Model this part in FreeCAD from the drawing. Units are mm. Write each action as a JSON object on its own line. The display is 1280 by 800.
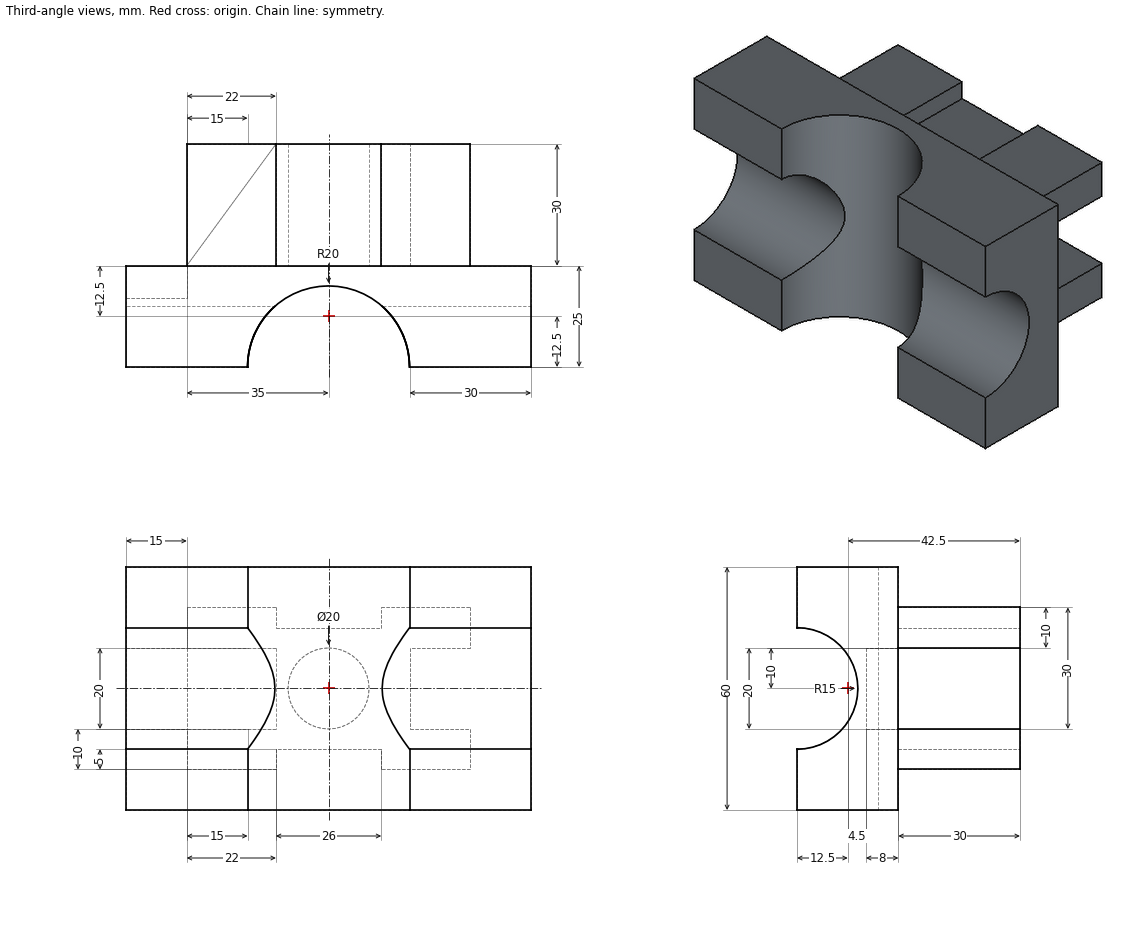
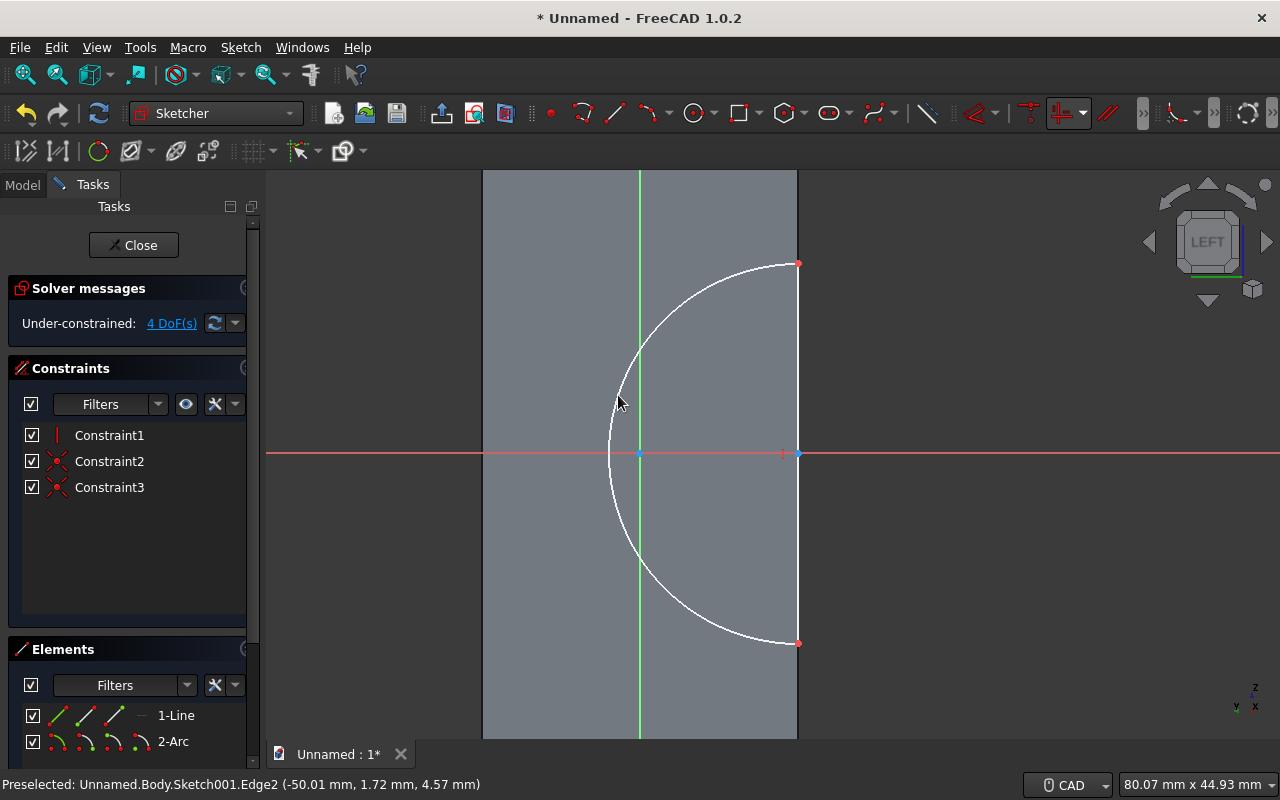
{"action": "left_click", "coordinate": [799, 454]}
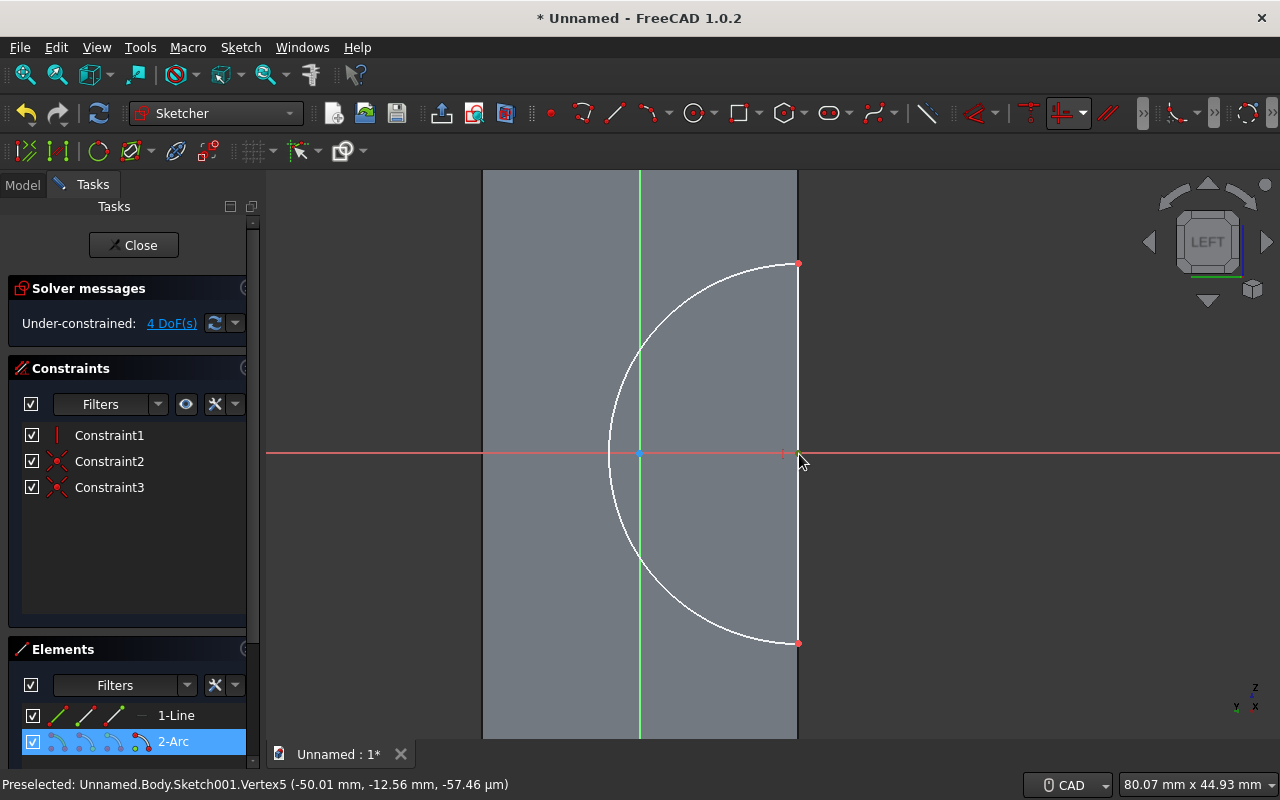
{"action": "left_click", "coordinate": [353, 453]}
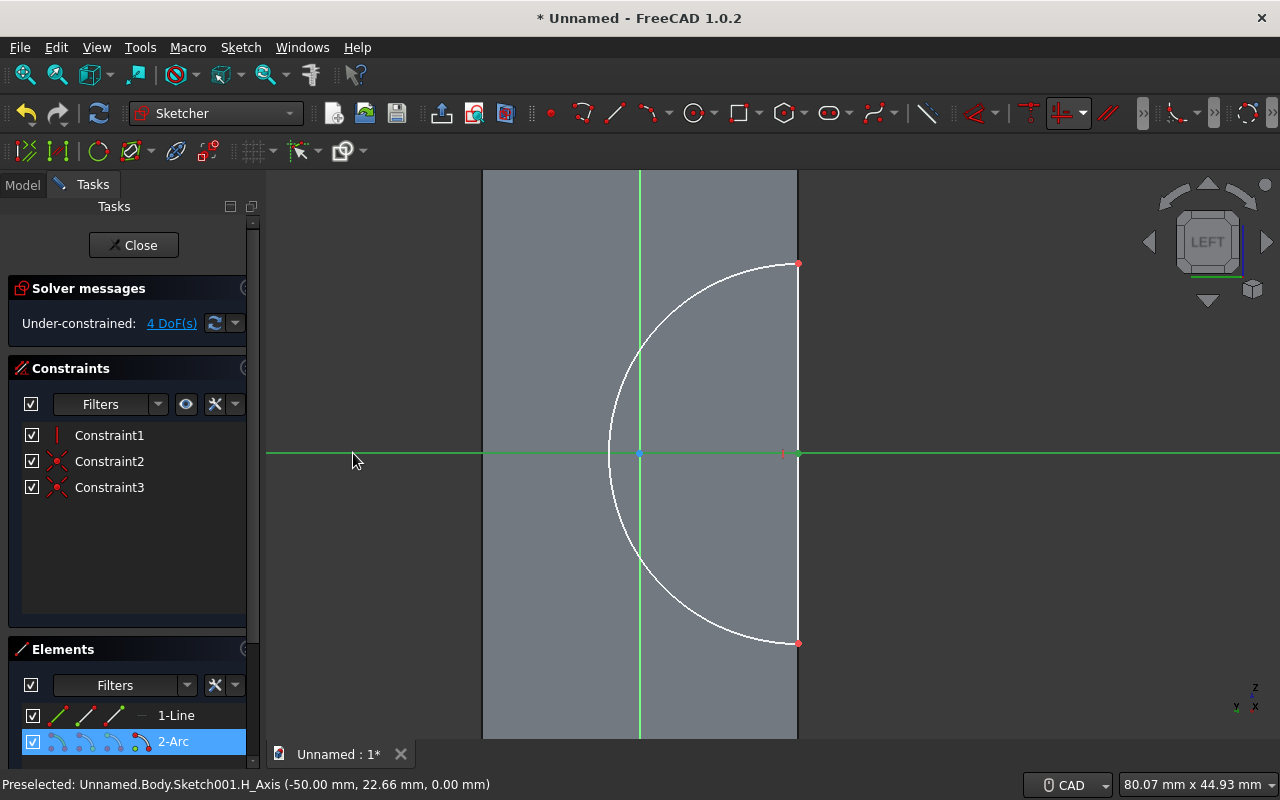
{"action": "key", "text": "c"}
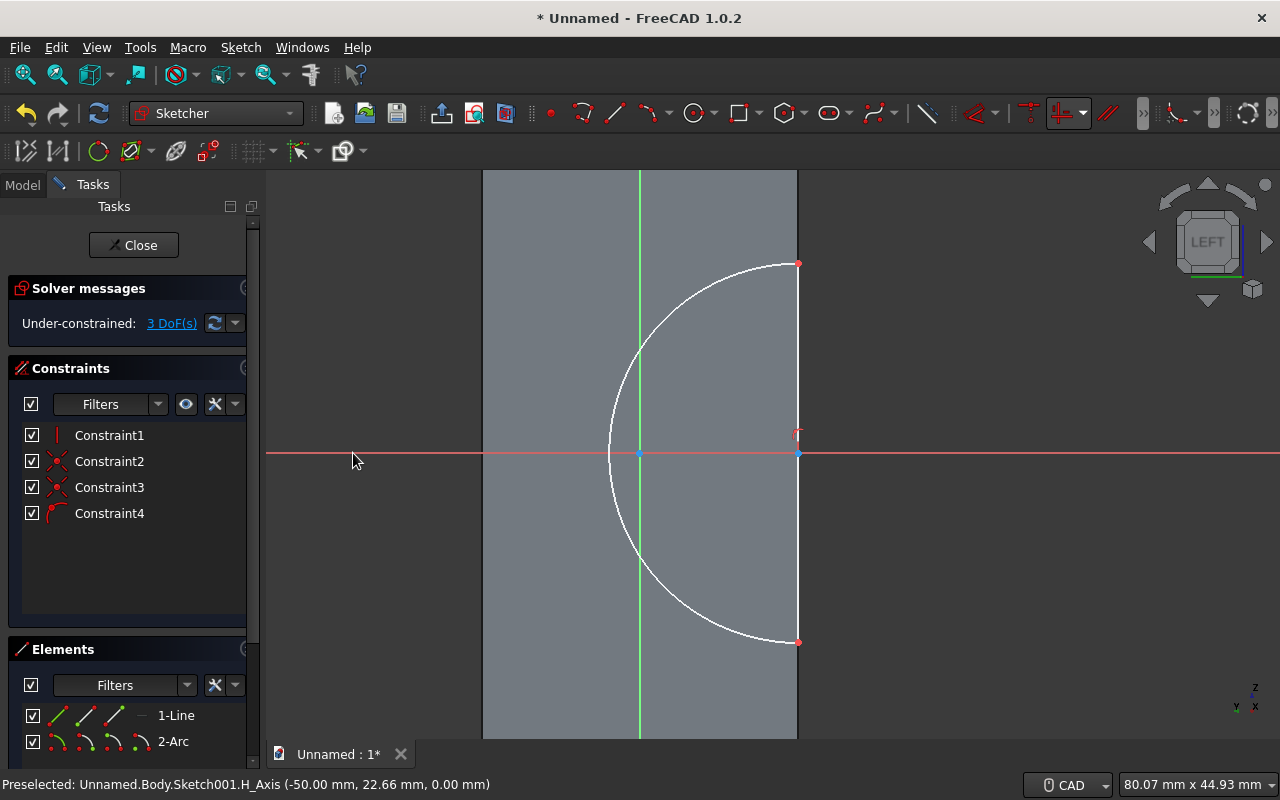
{"action": "left_click", "coordinate": [974, 114]}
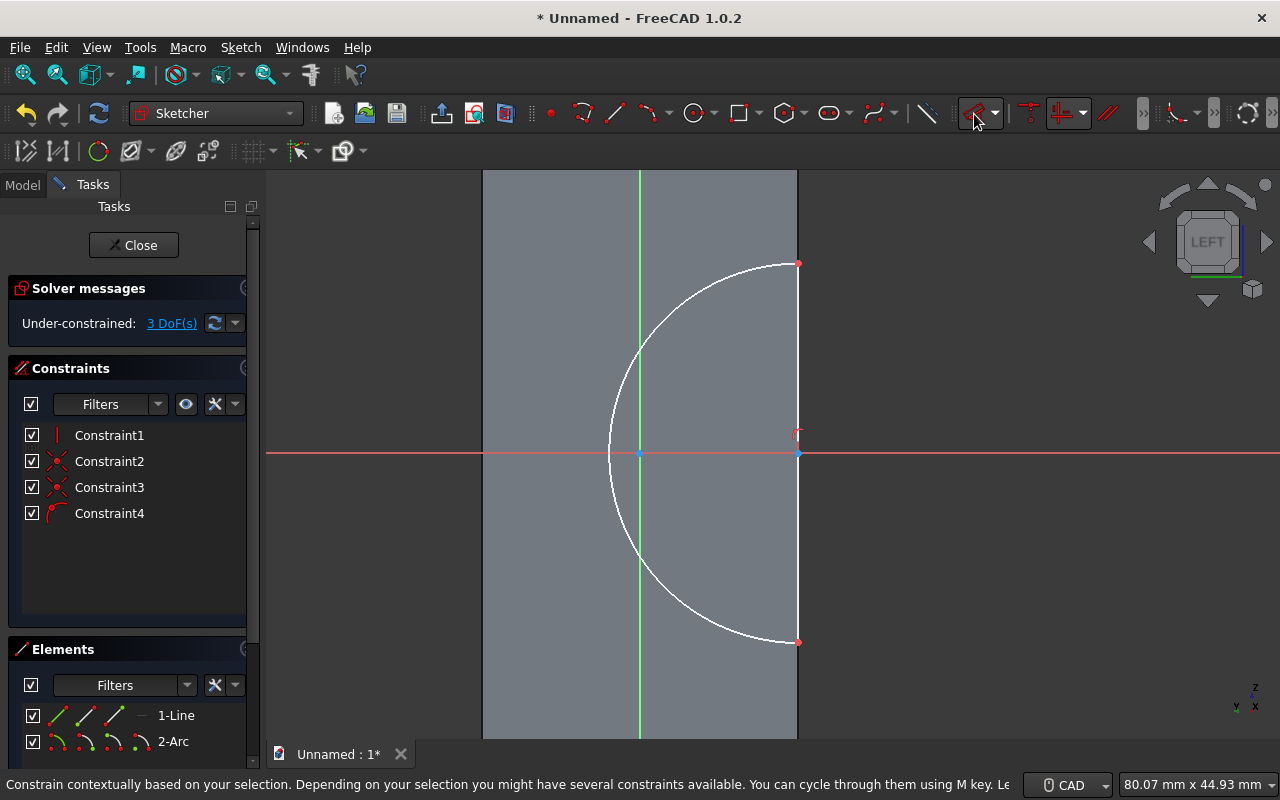
{"action": "left_click", "coordinate": [609, 453]}
{"action": "left_click", "coordinate": [604, 347]}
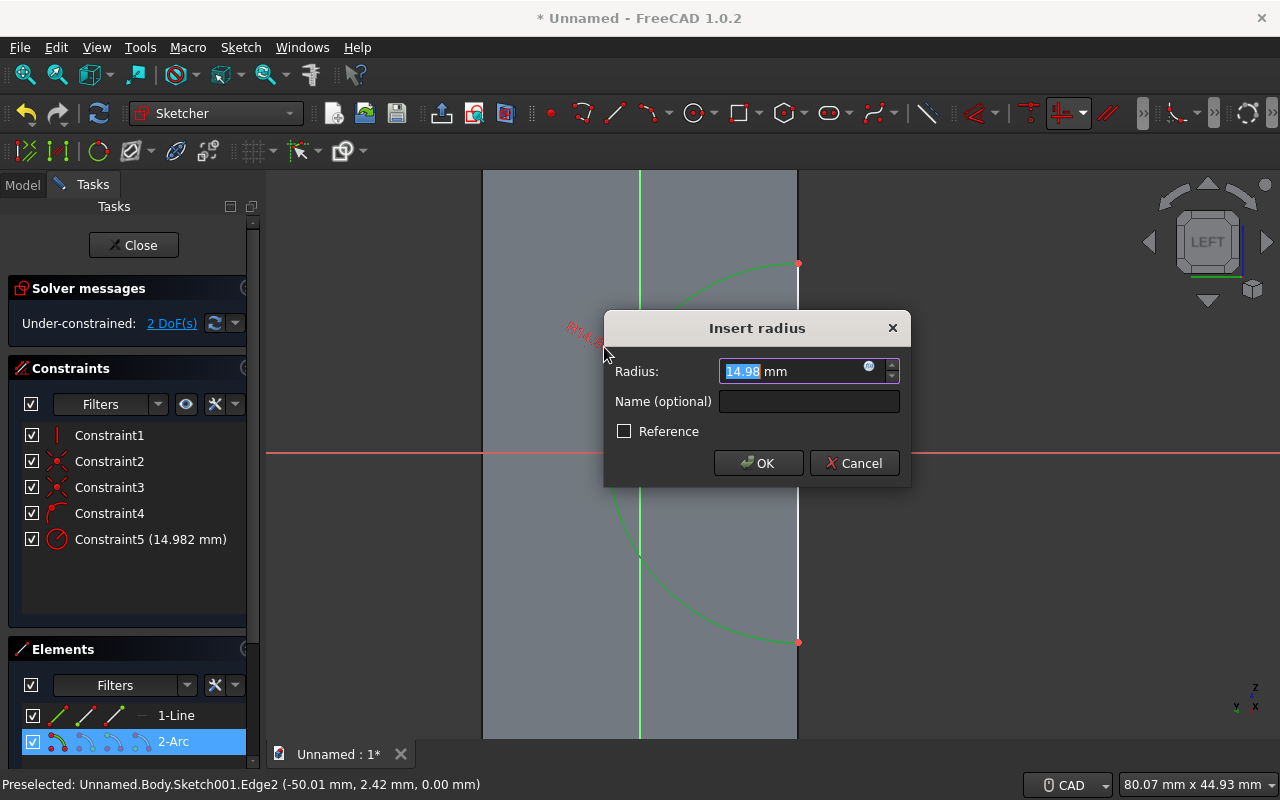
{"action": "type", "text": "15"}
{"action": "key", "text": "Return"}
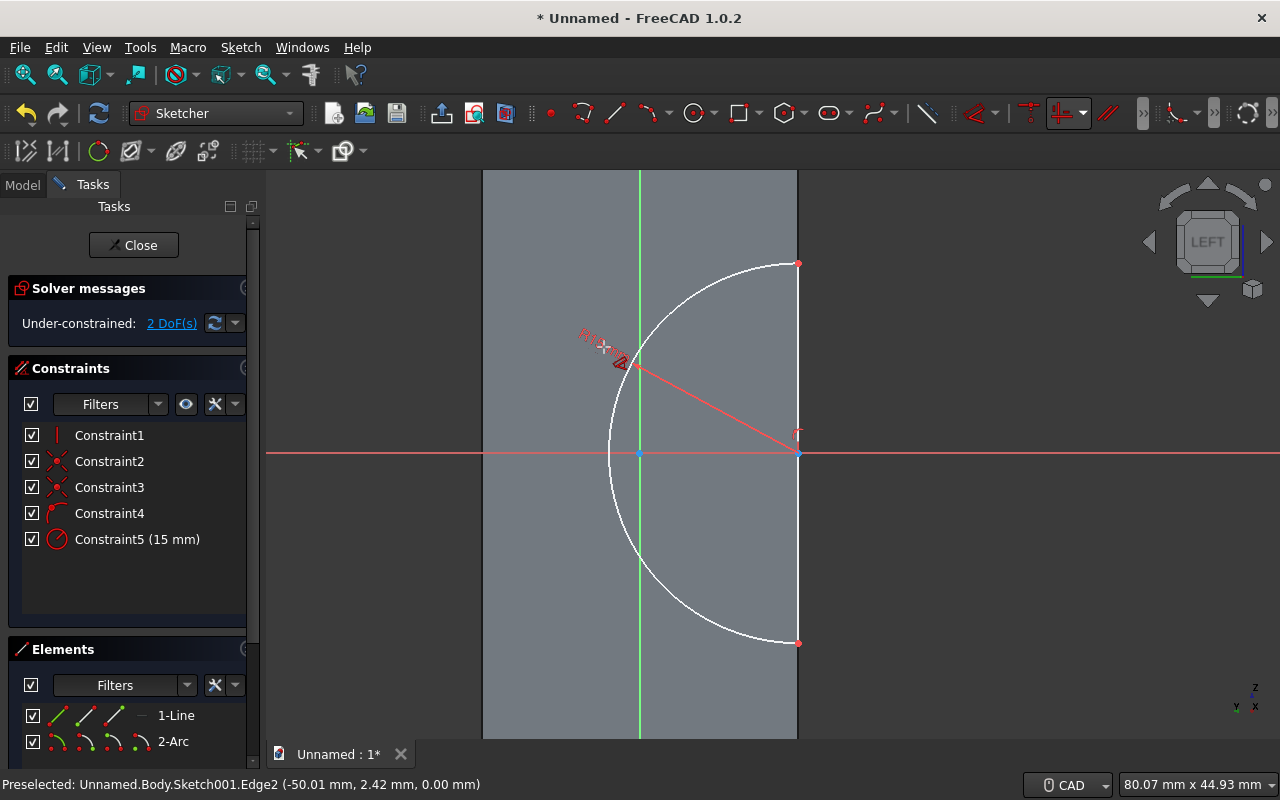
{"action": "left_click", "coordinate": [798, 643]}
{"action": "left_click", "coordinate": [719, 677]}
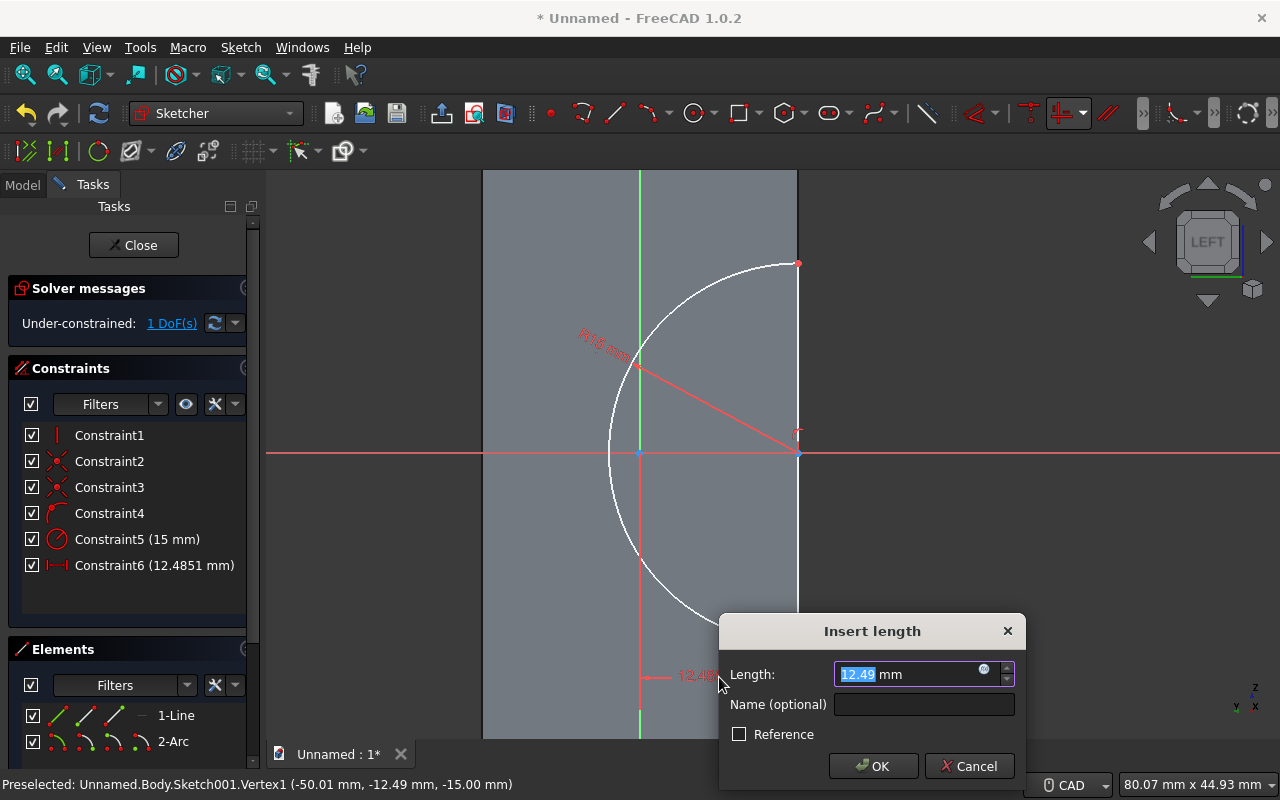
{"action": "type", "text": "12.5"}
{"action": "key", "text": "Return"}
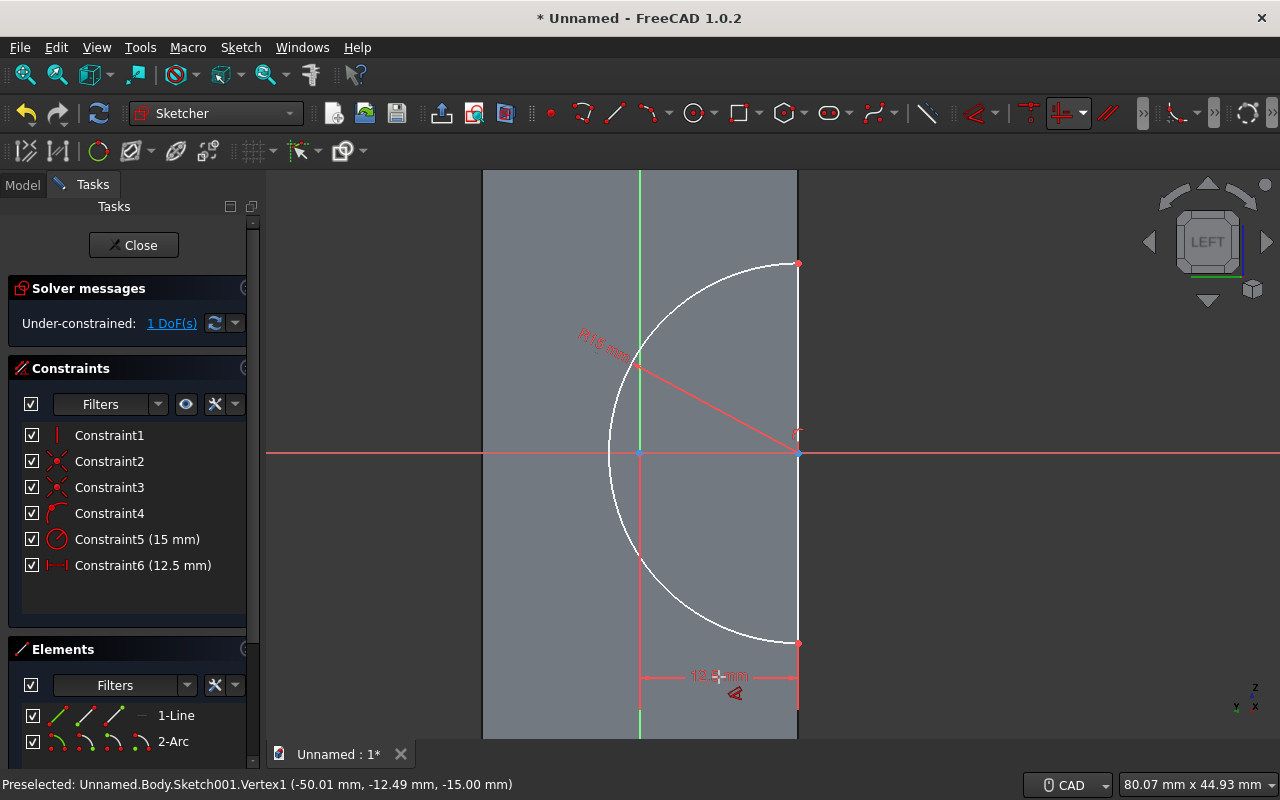
{"action": "left_click", "coordinate": [799, 453]}
{"action": "left_click", "coordinate": [719, 487]}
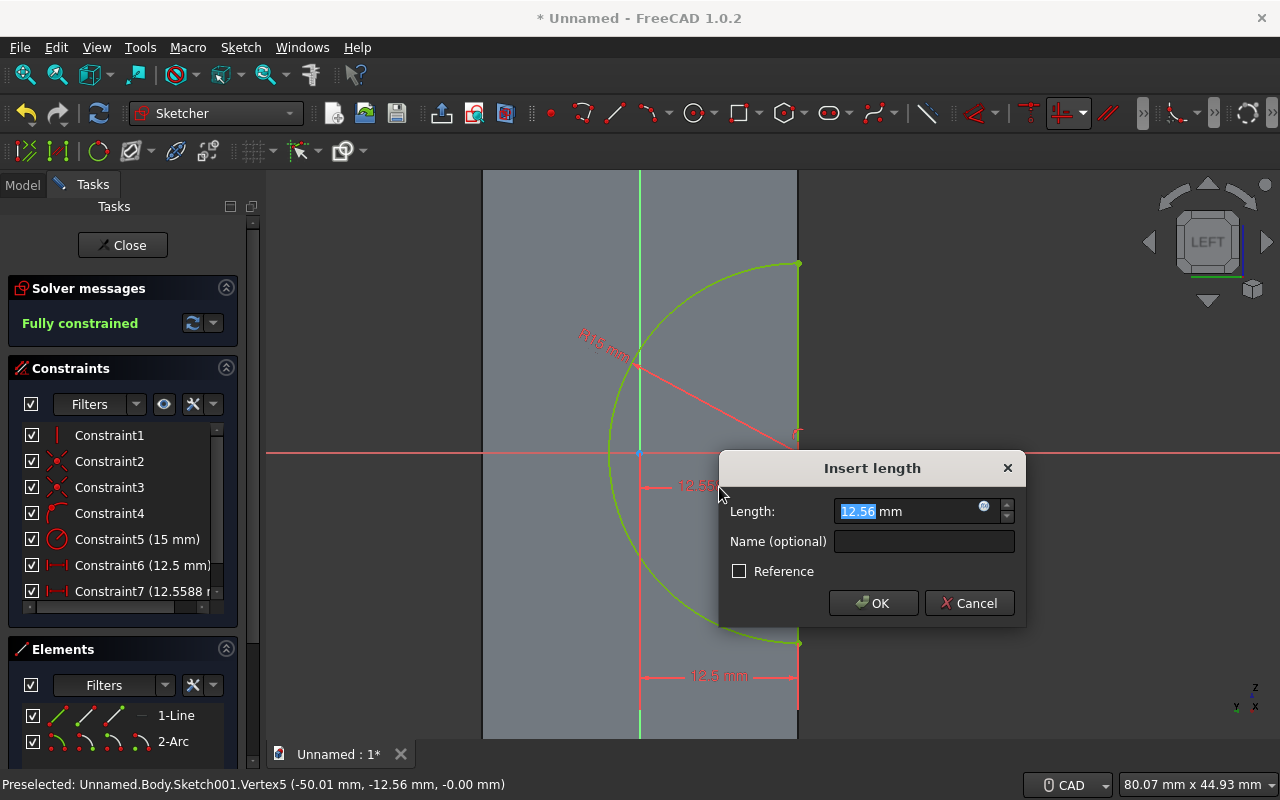
{"action": "type", "text": "12.5"}
{"action": "key", "text": "Return"}
{"action": "key", "text": "Escape"}